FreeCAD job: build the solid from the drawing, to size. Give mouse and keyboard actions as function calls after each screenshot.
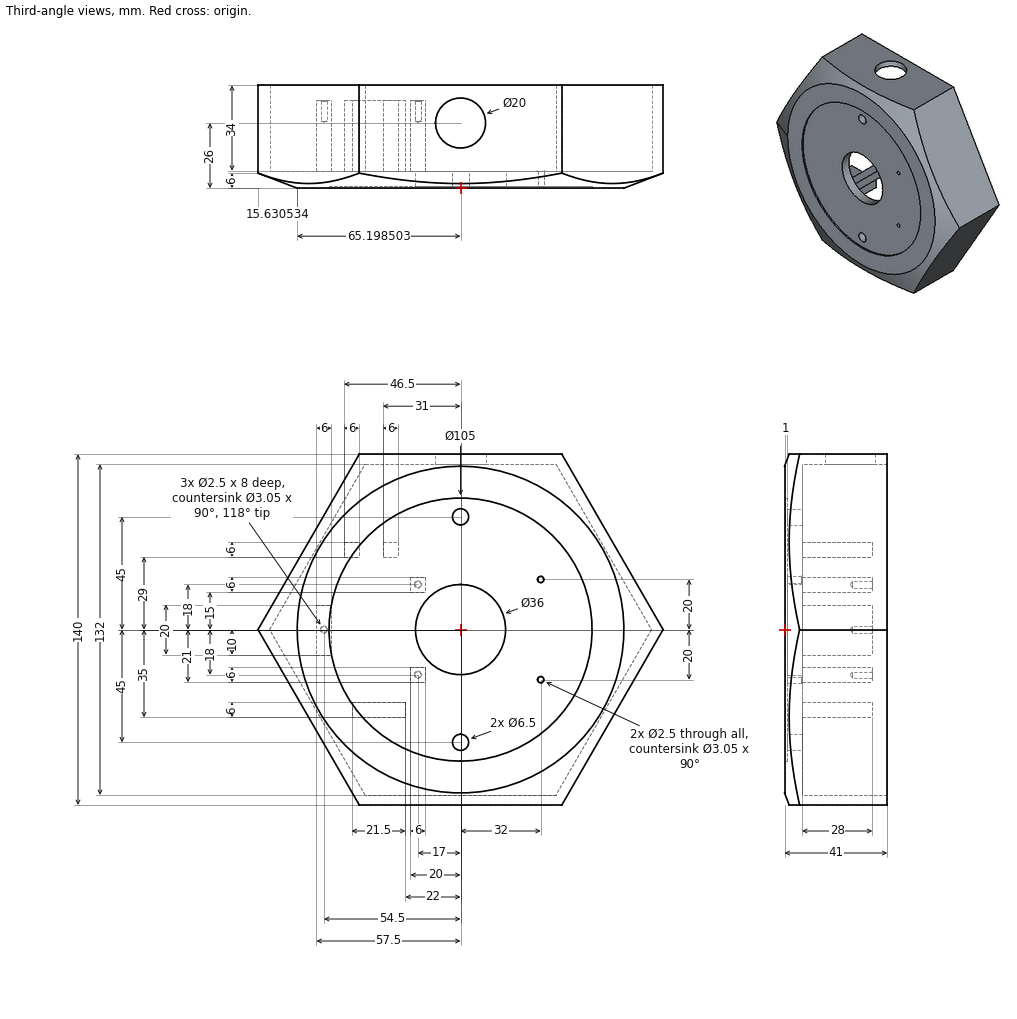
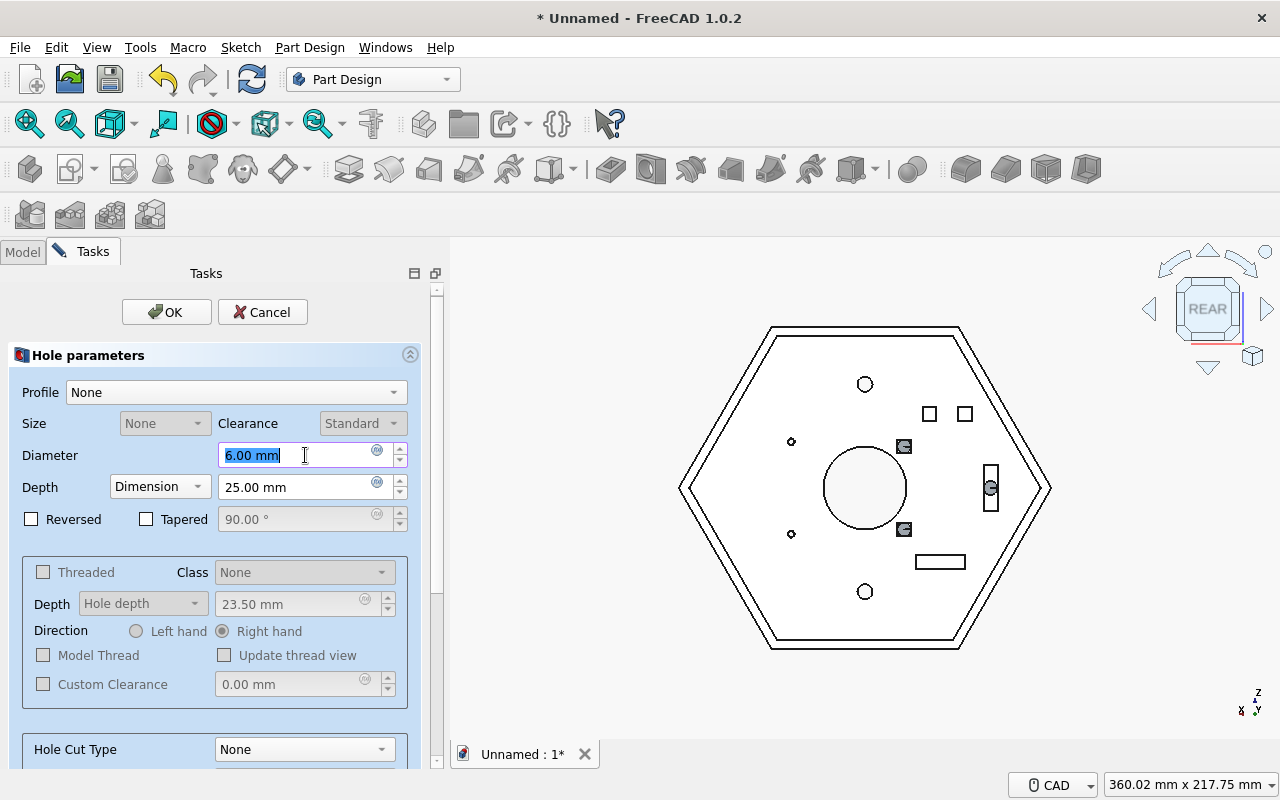
text(2.5)
key(Tab)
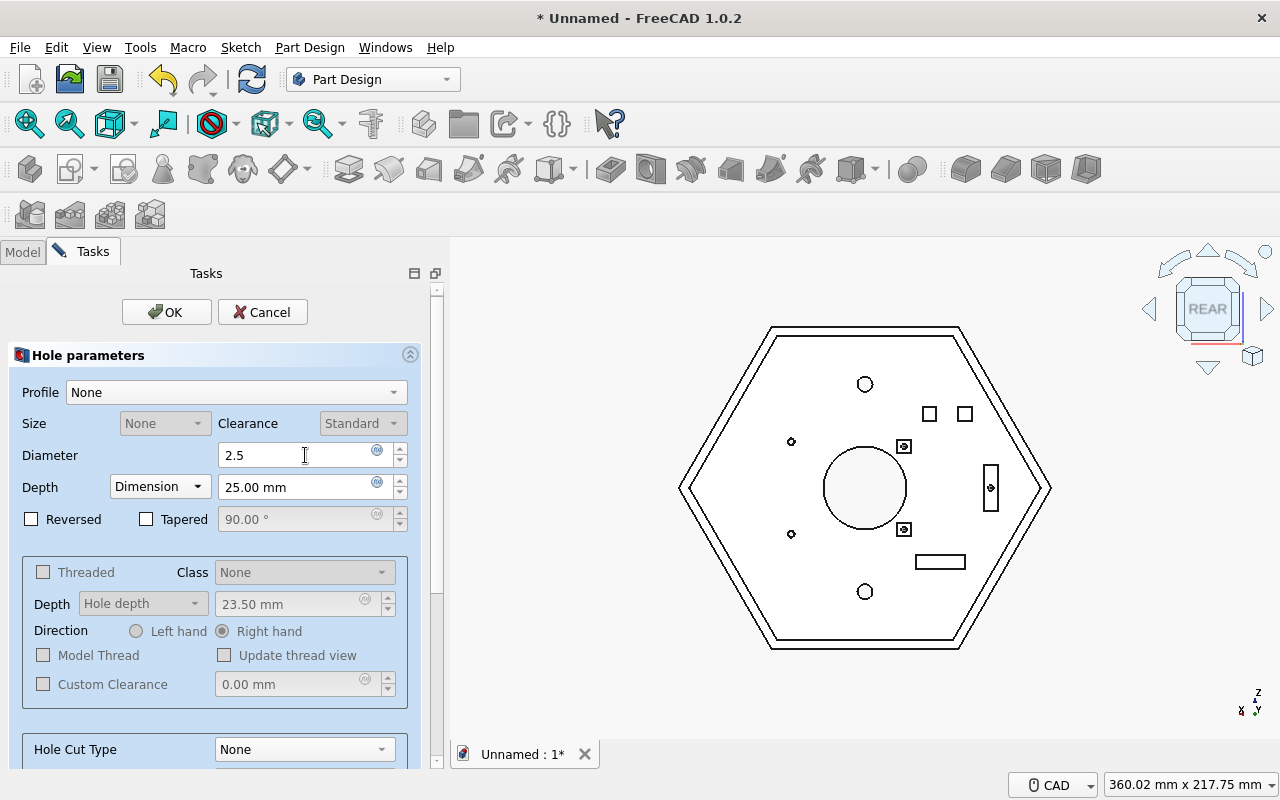
triple_click(305, 487)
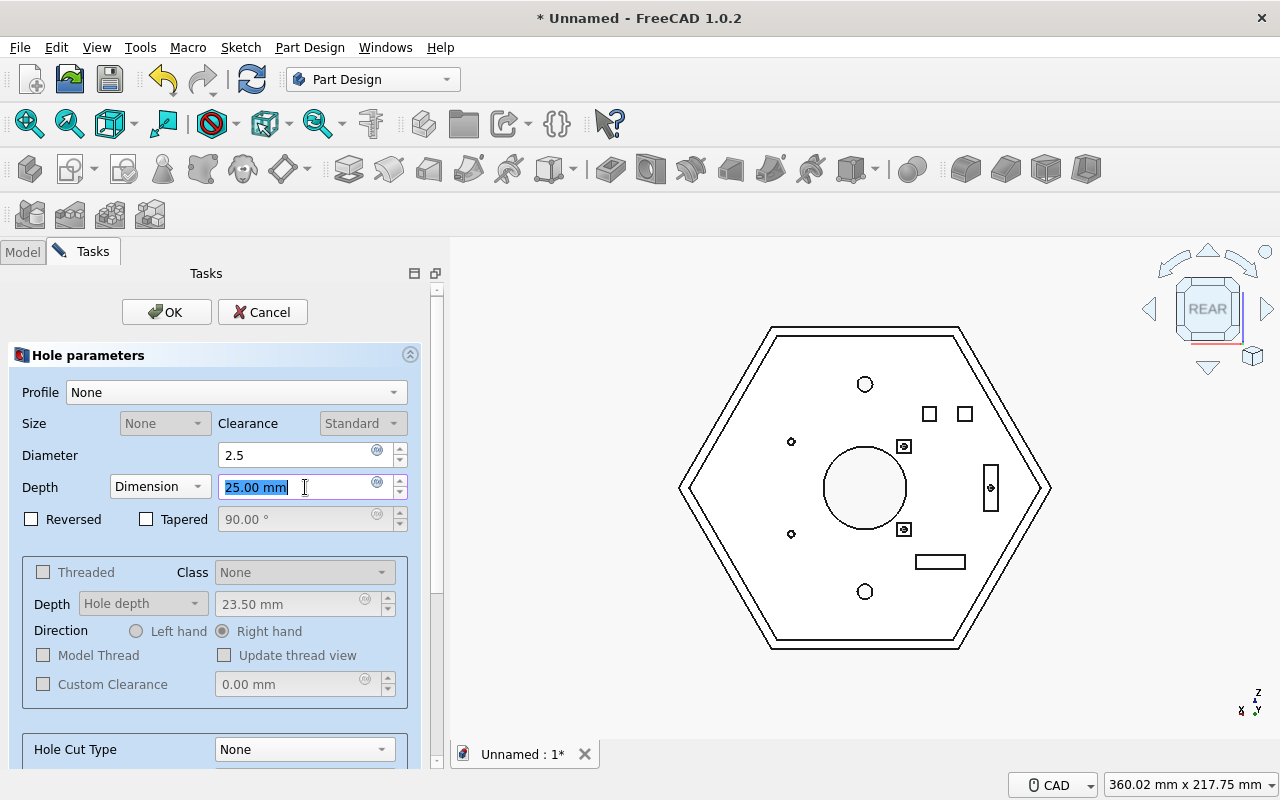
text(8)
key(Tab)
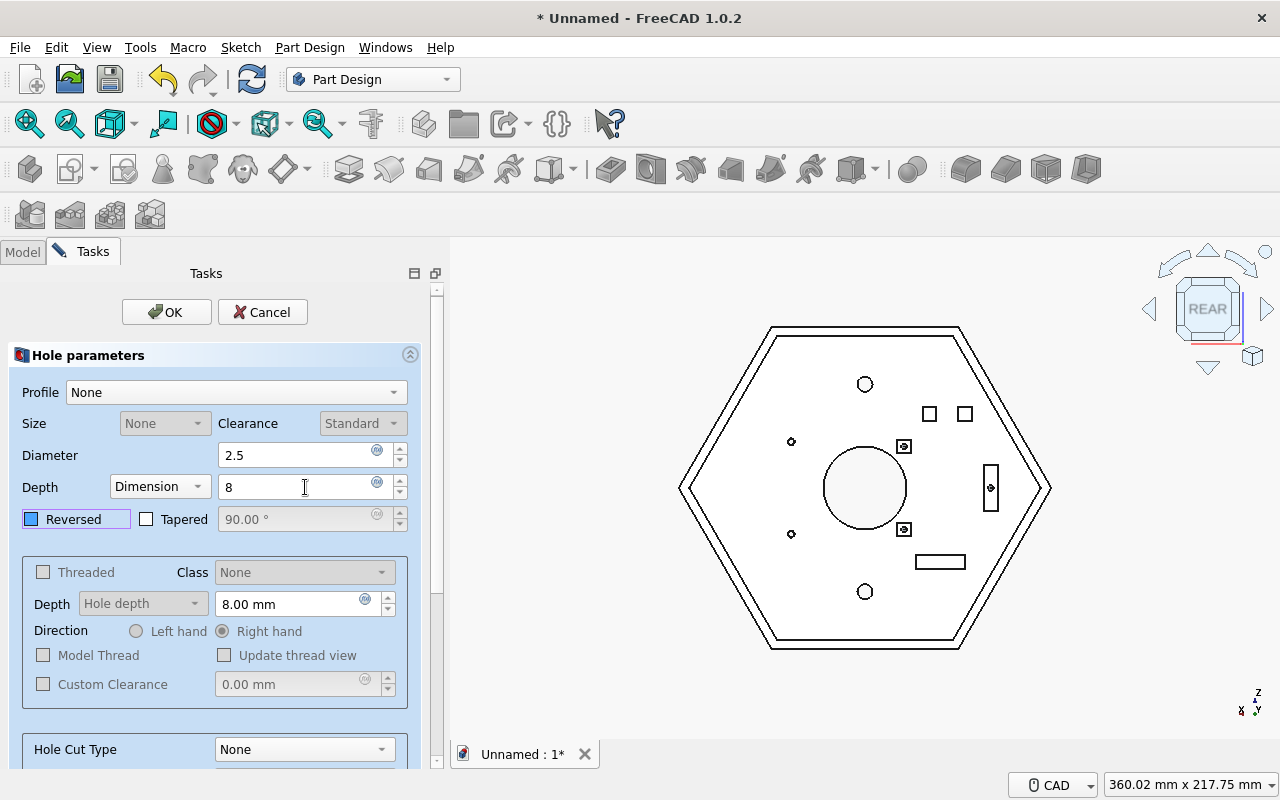
click(306, 750)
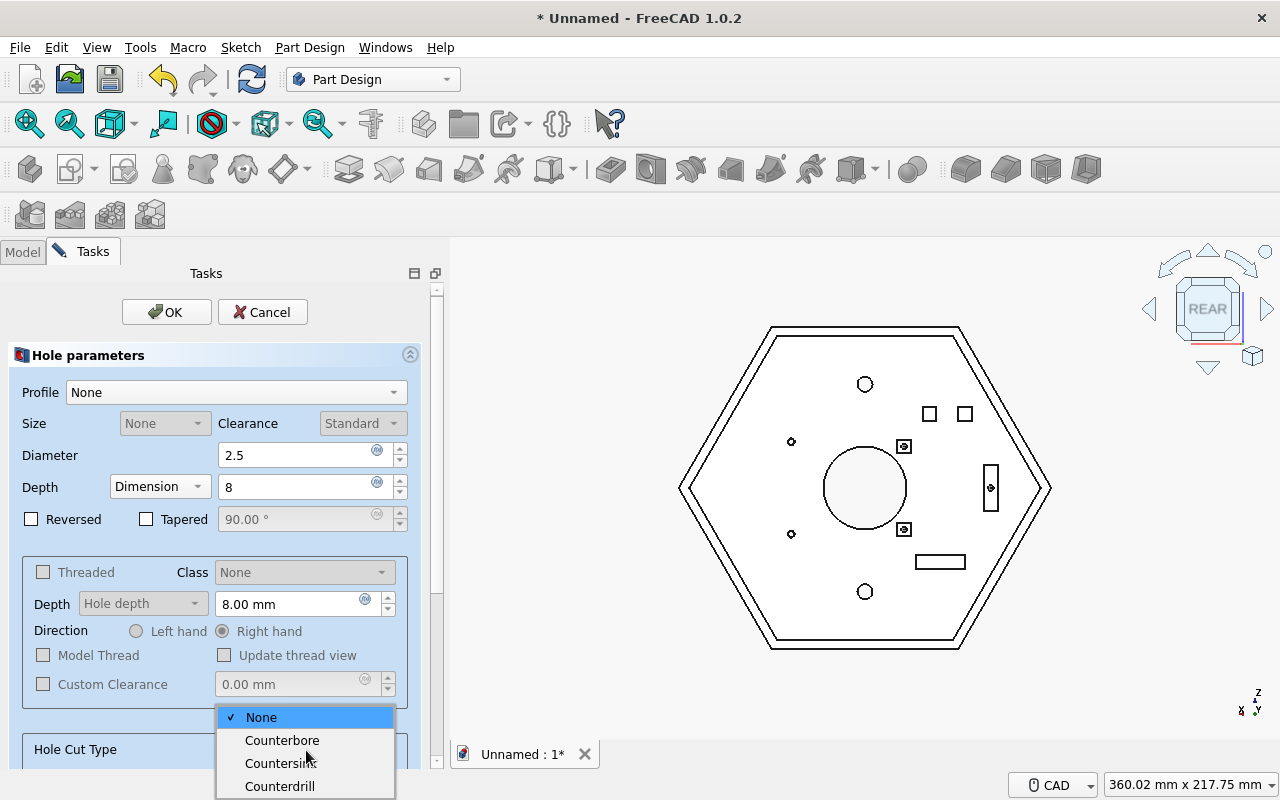
click(304, 764)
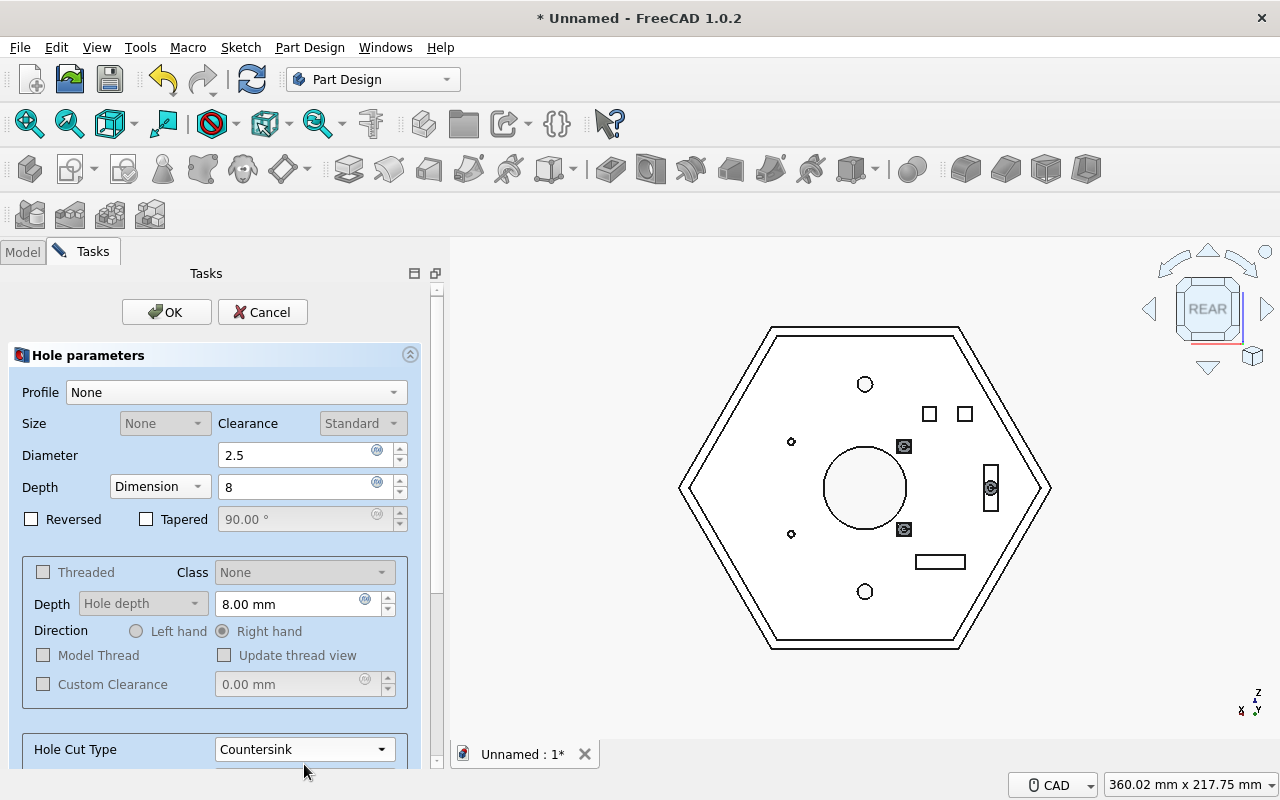
scroll(437, 526, down, 2)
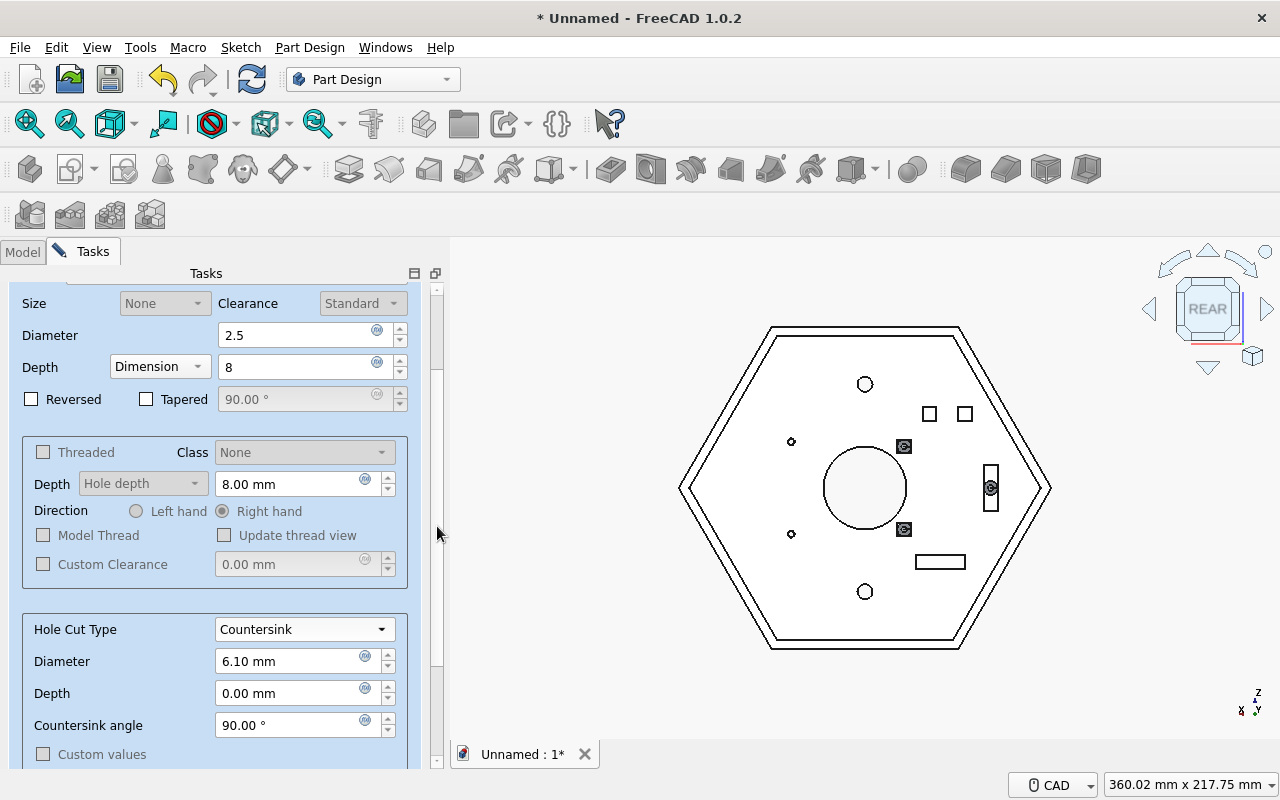
triple_click(298, 661)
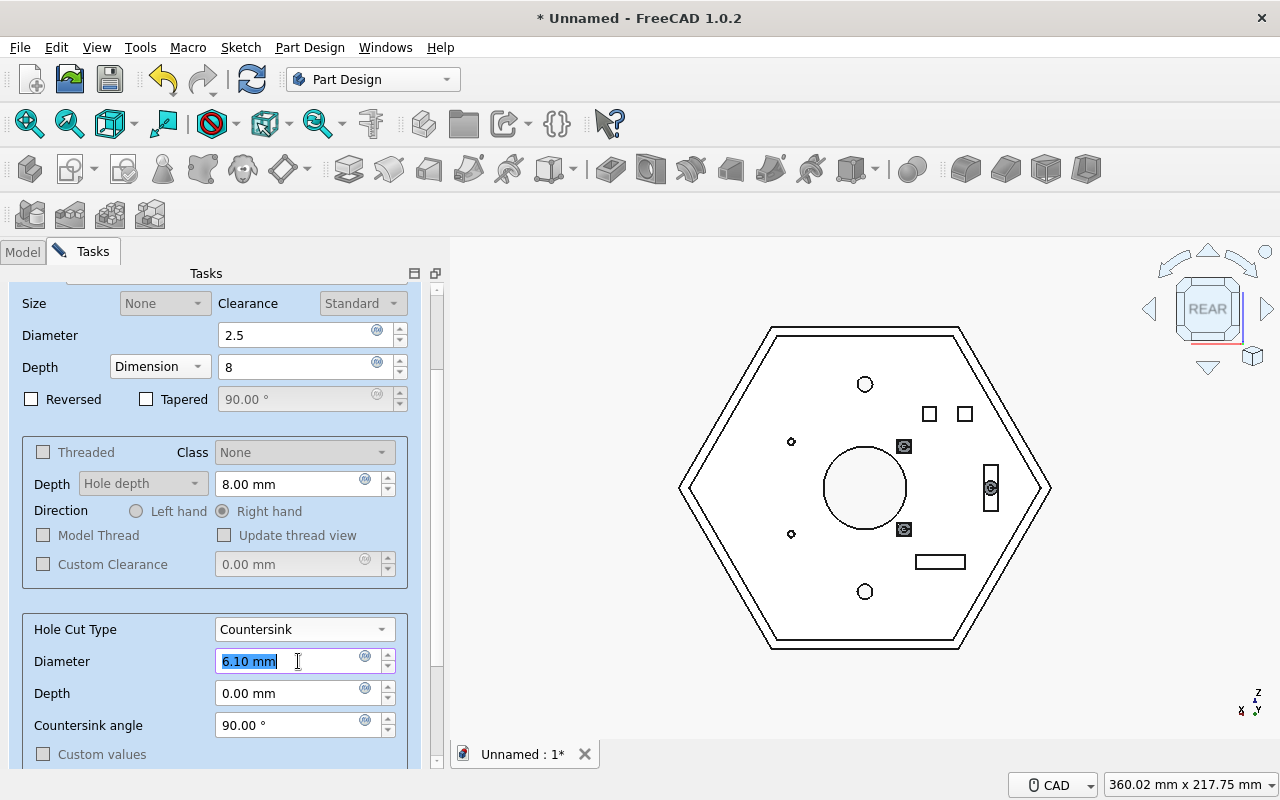
text(3.05)
key(Tab)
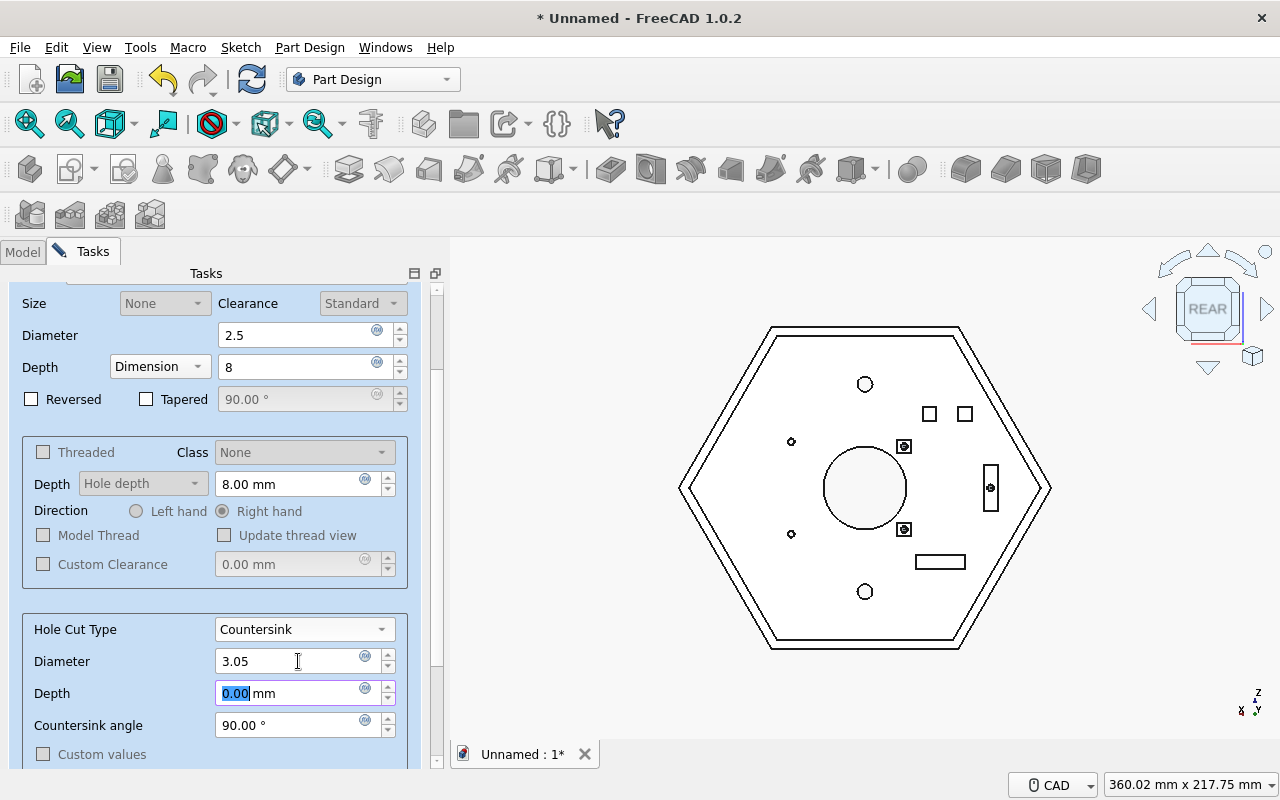
scroll(437, 526, up, 3)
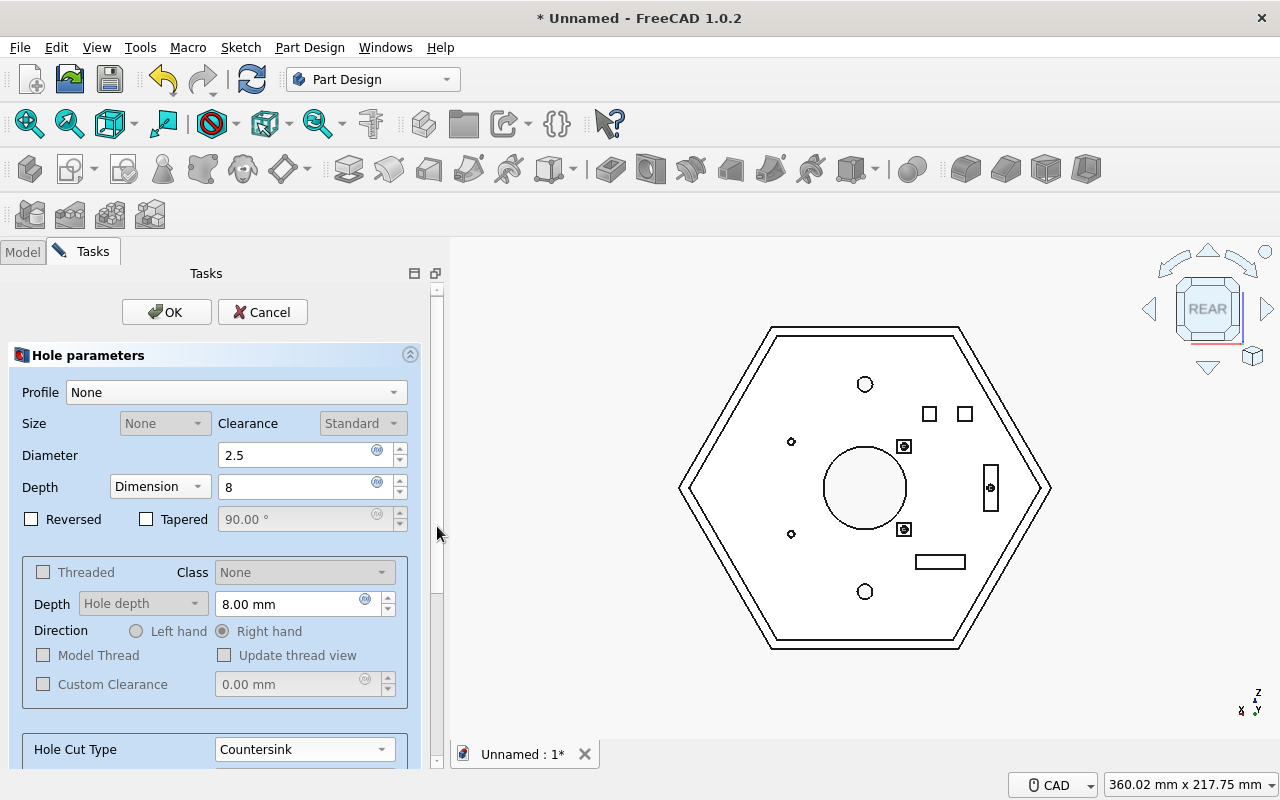
click(167, 312)